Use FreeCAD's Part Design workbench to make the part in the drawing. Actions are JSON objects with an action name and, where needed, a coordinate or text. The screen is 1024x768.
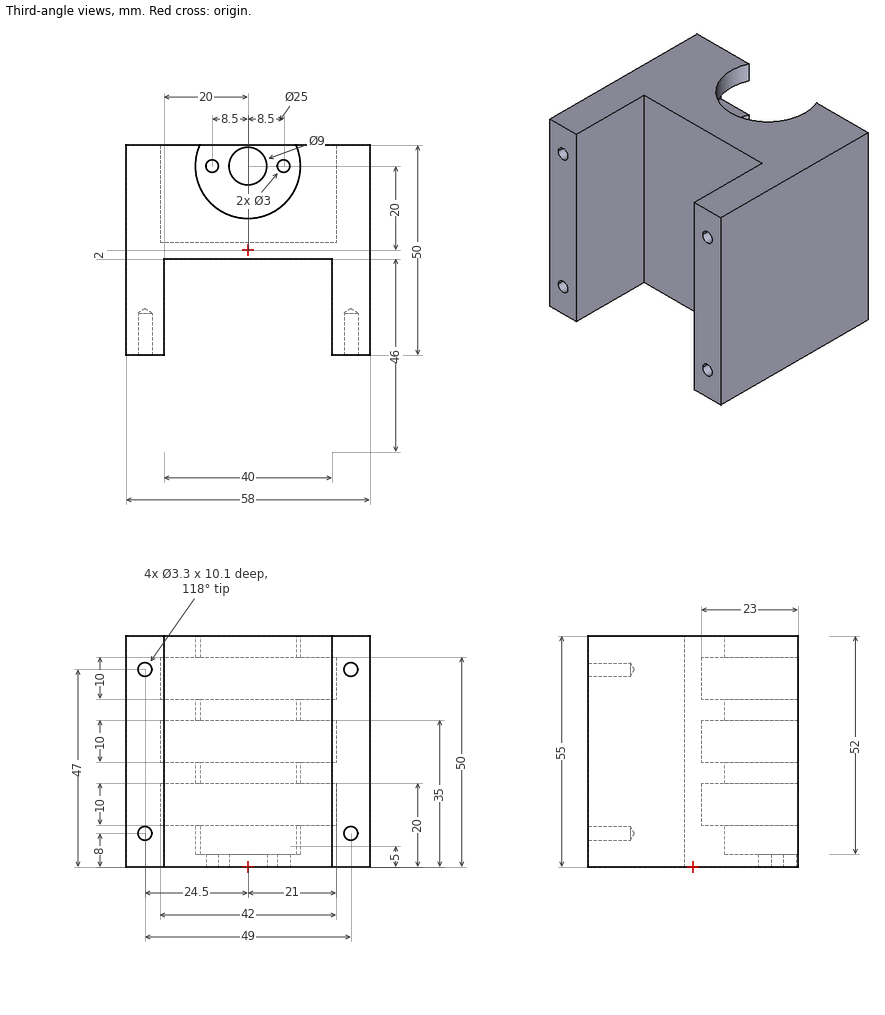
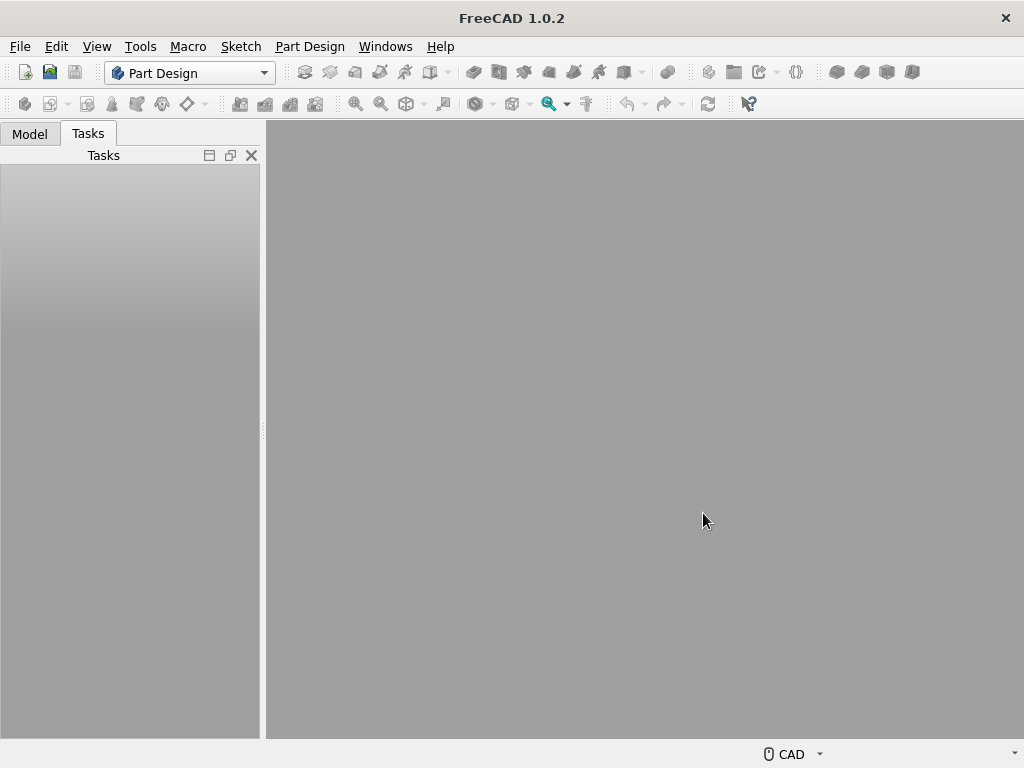
{"action": "left_click", "coordinate": [25, 72]}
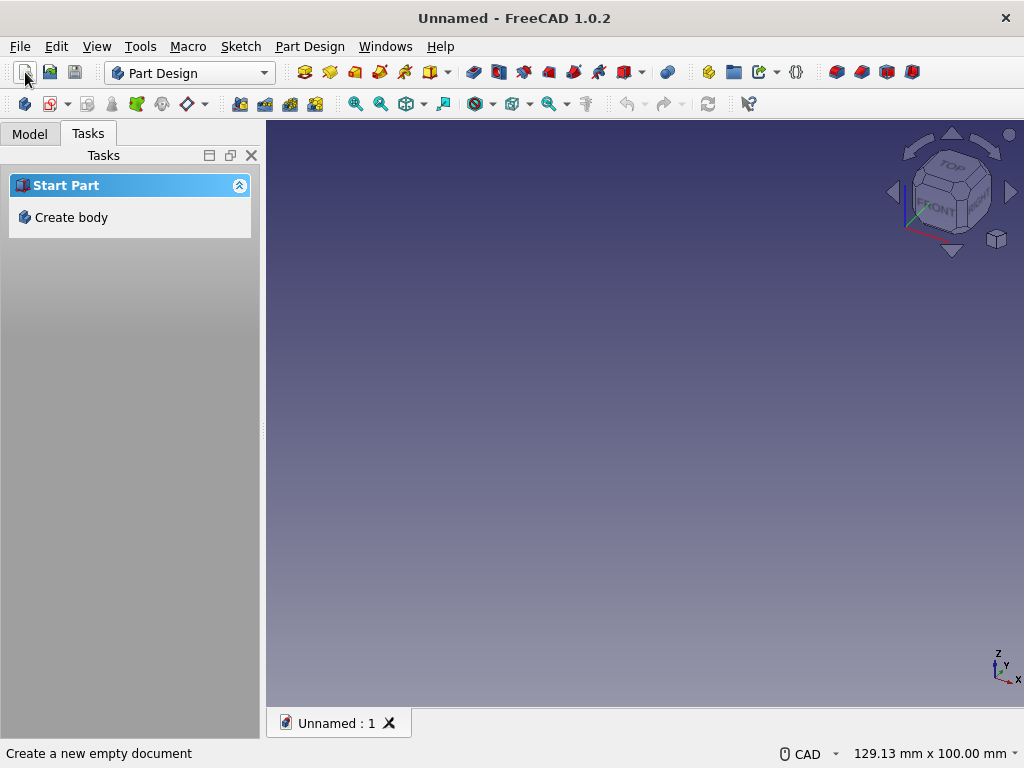
{"action": "left_click", "coordinate": [50, 104]}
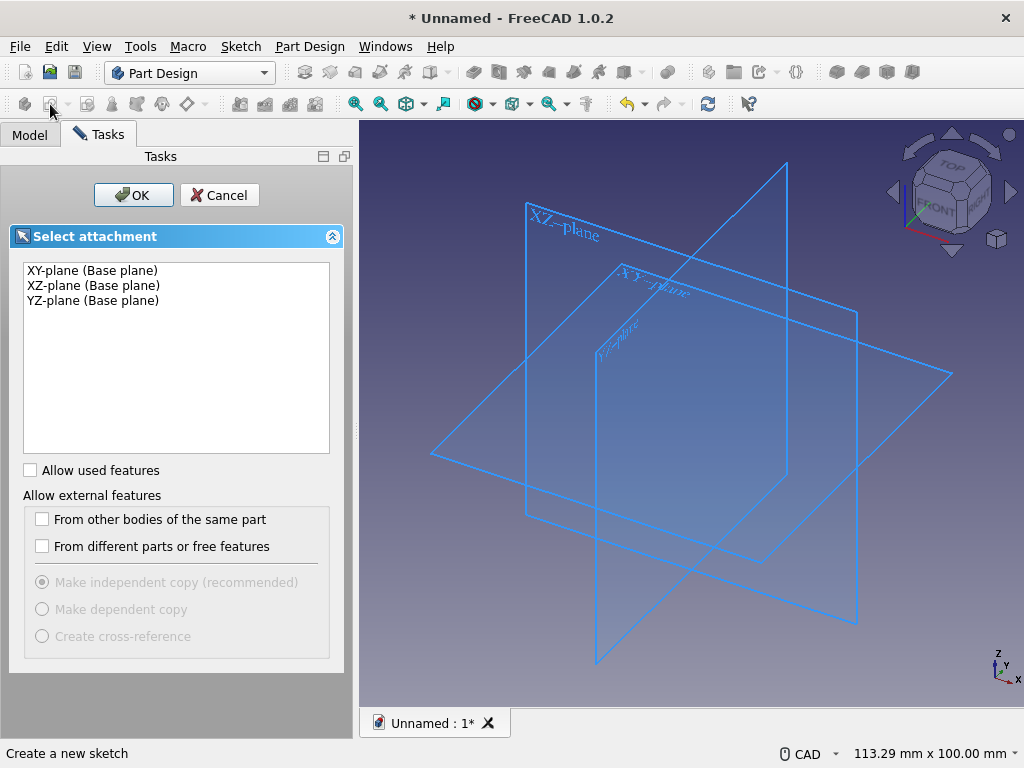
{"action": "left_click", "coordinate": [84, 270]}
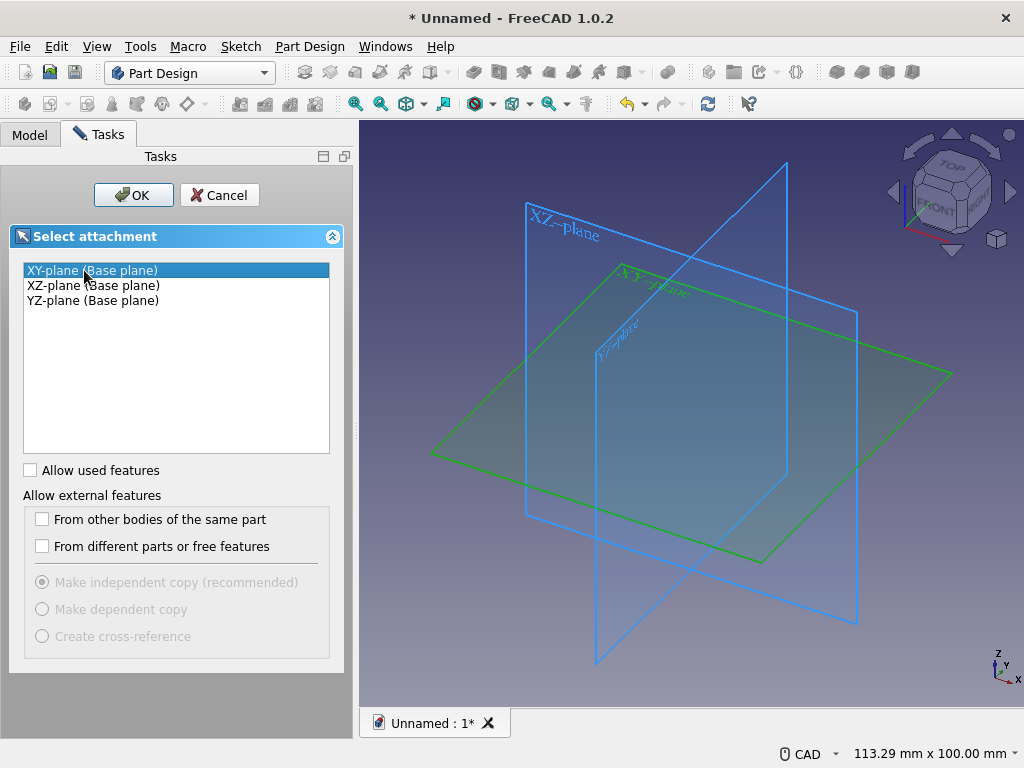
{"action": "left_click", "coordinate": [134, 195]}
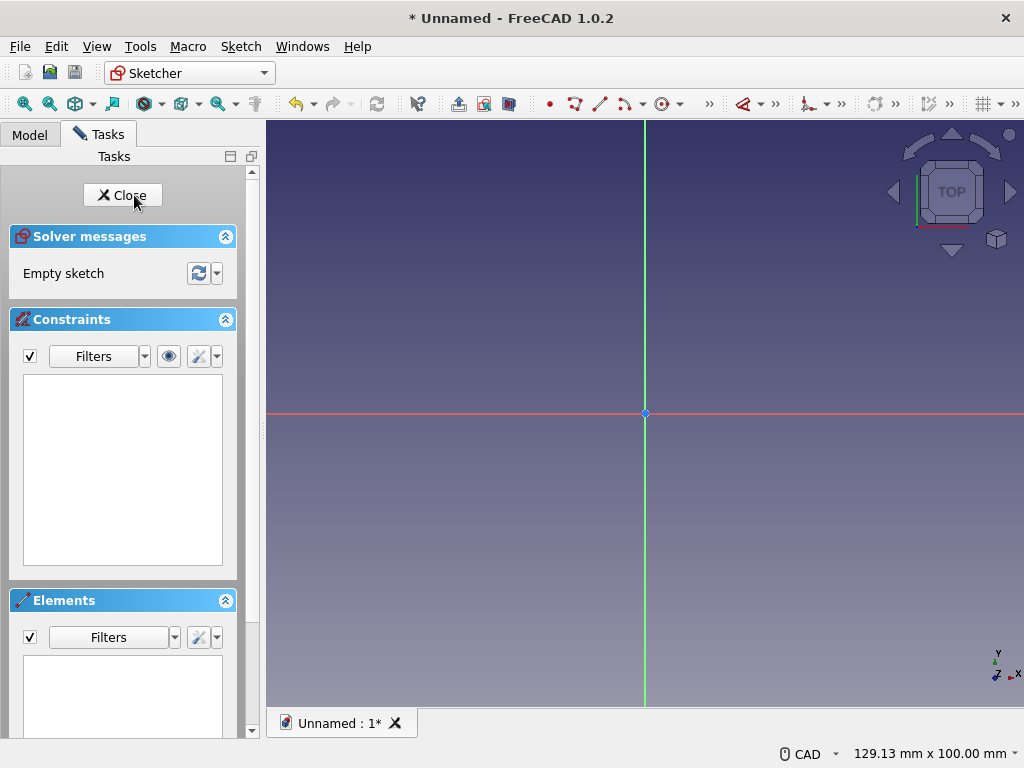
{"action": "key", "text": "g v"}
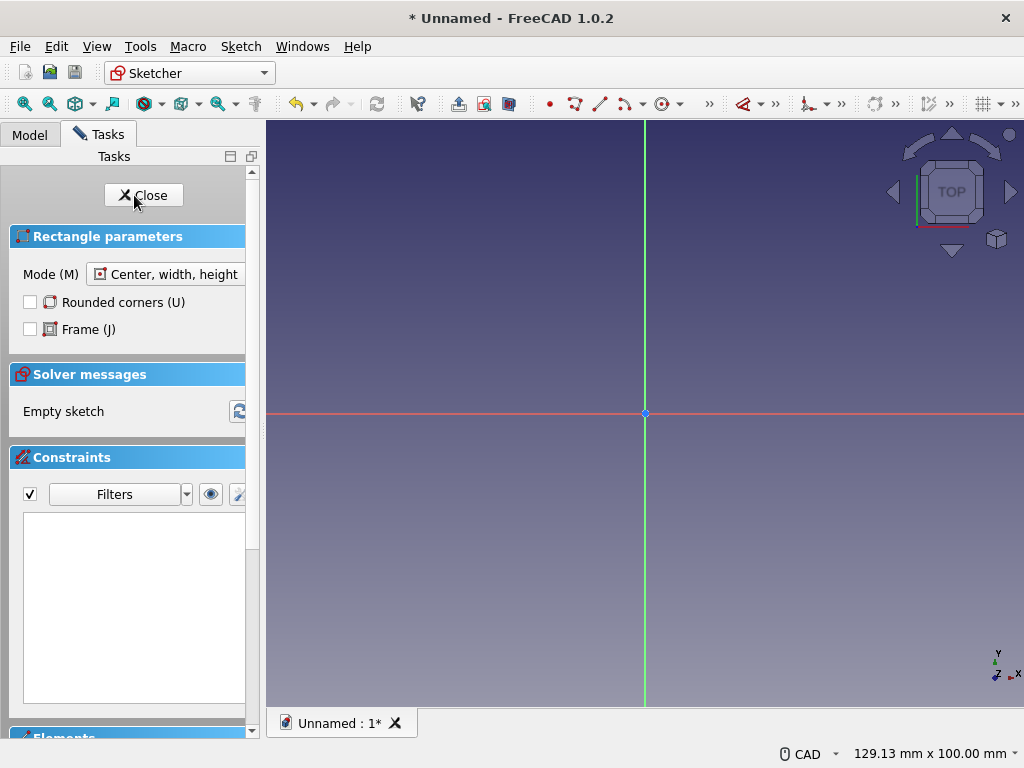
{"action": "left_click", "coordinate": [645, 414]}
{"action": "mouse_move", "coordinate": [815, 267]}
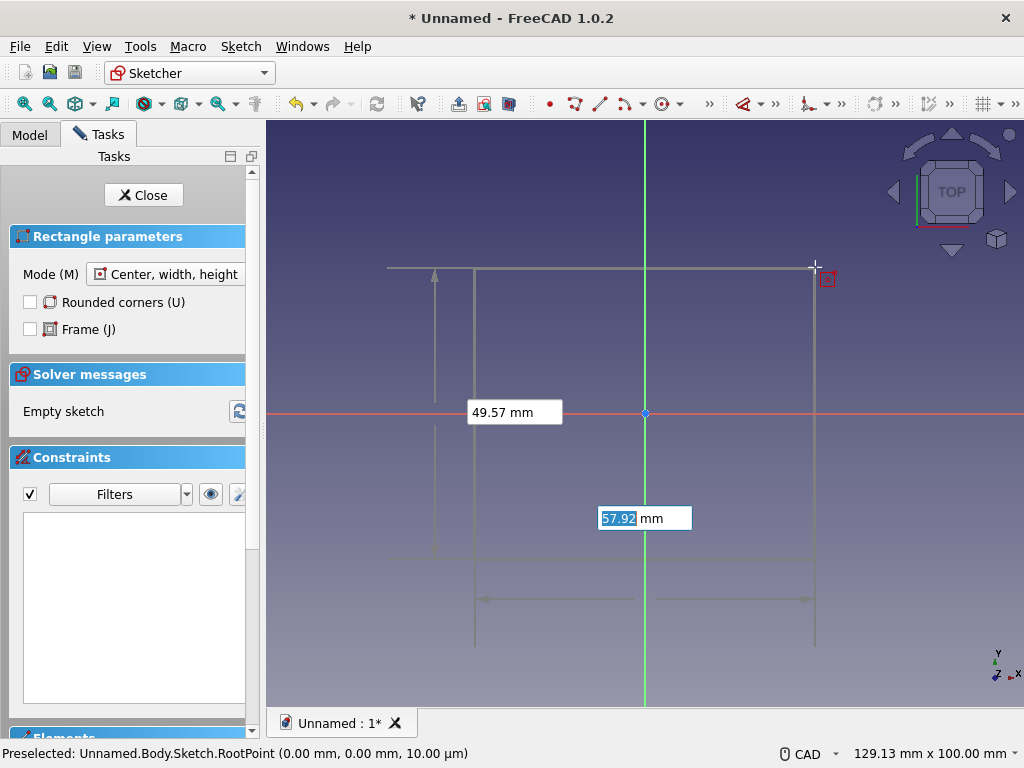
{"action": "type", "text": "58"}
{"action": "key", "text": "Tab"}
{"action": "type", "text": "50"}
{"action": "key", "text": "Return"}
{"action": "key", "text": "Escape"}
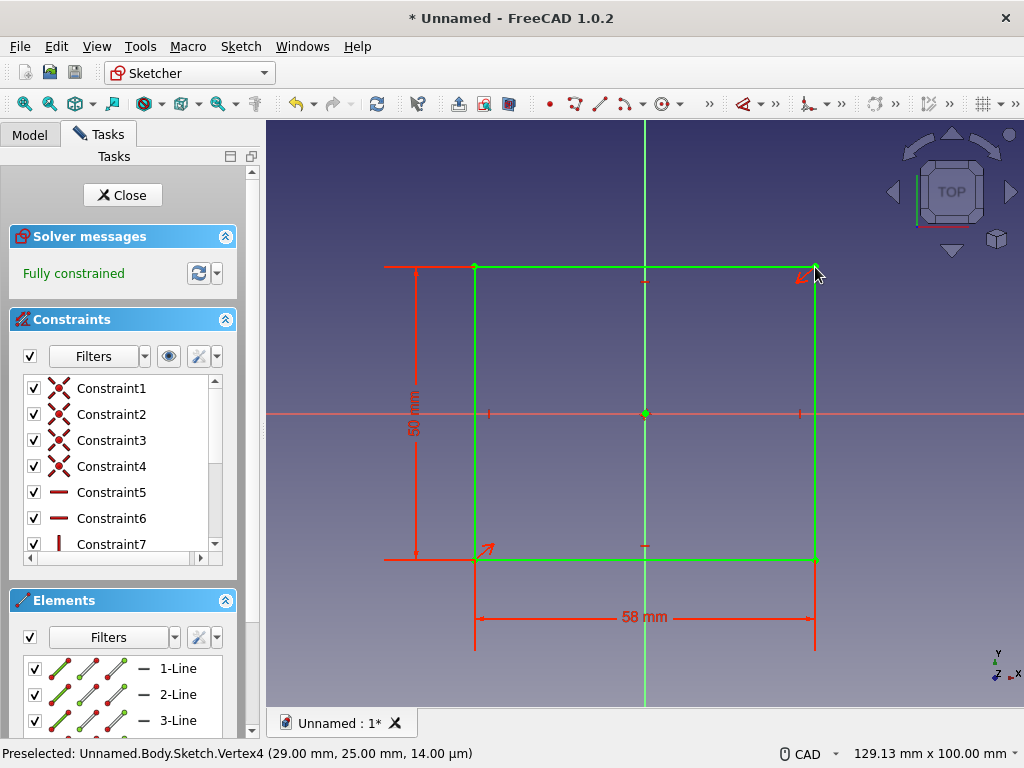
{"action": "left_click", "coordinate": [123, 195]}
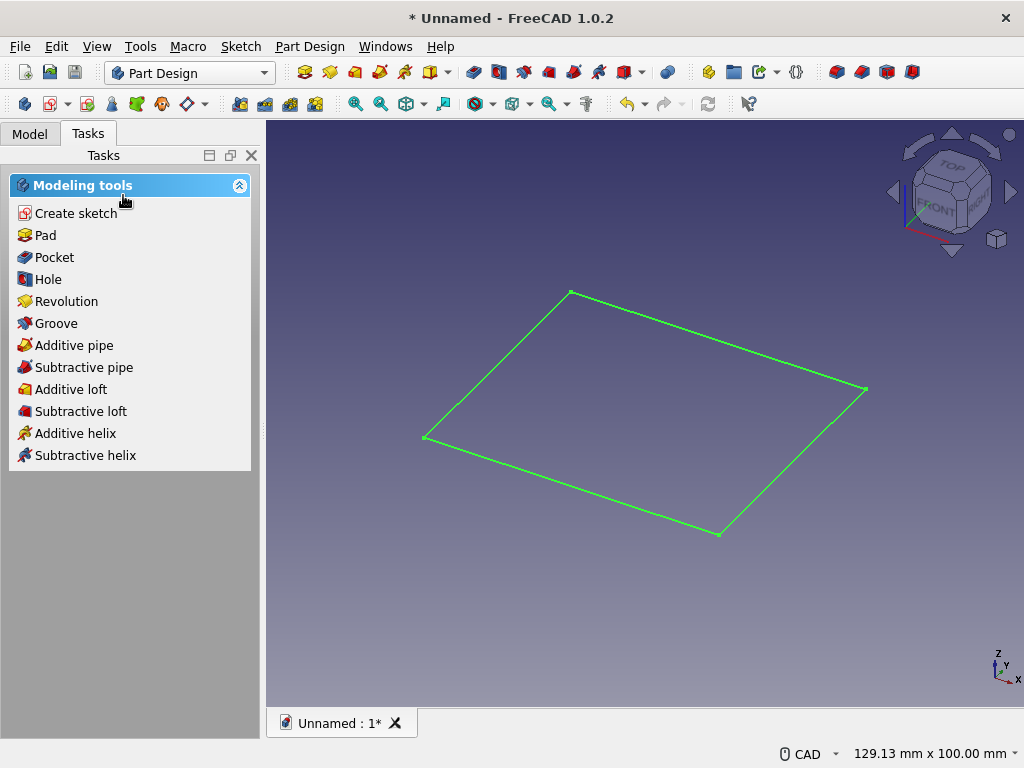
{"action": "left_click", "coordinate": [305, 72]}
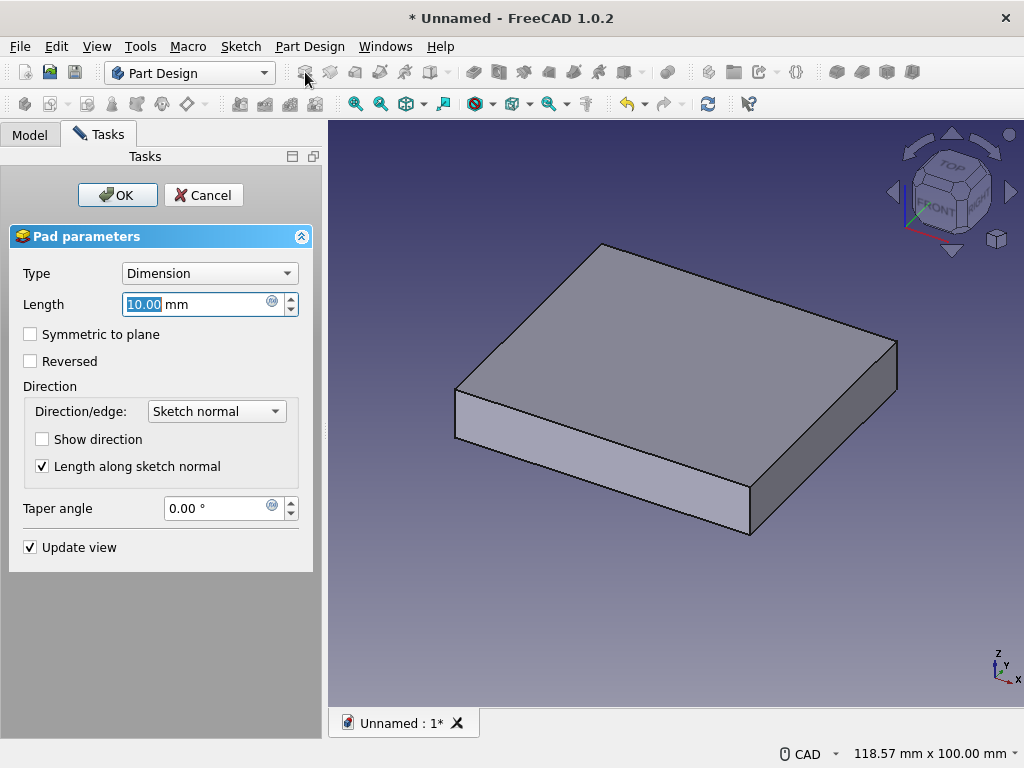
{"action": "type", "text": "55"}
{"action": "key", "text": "Tab"}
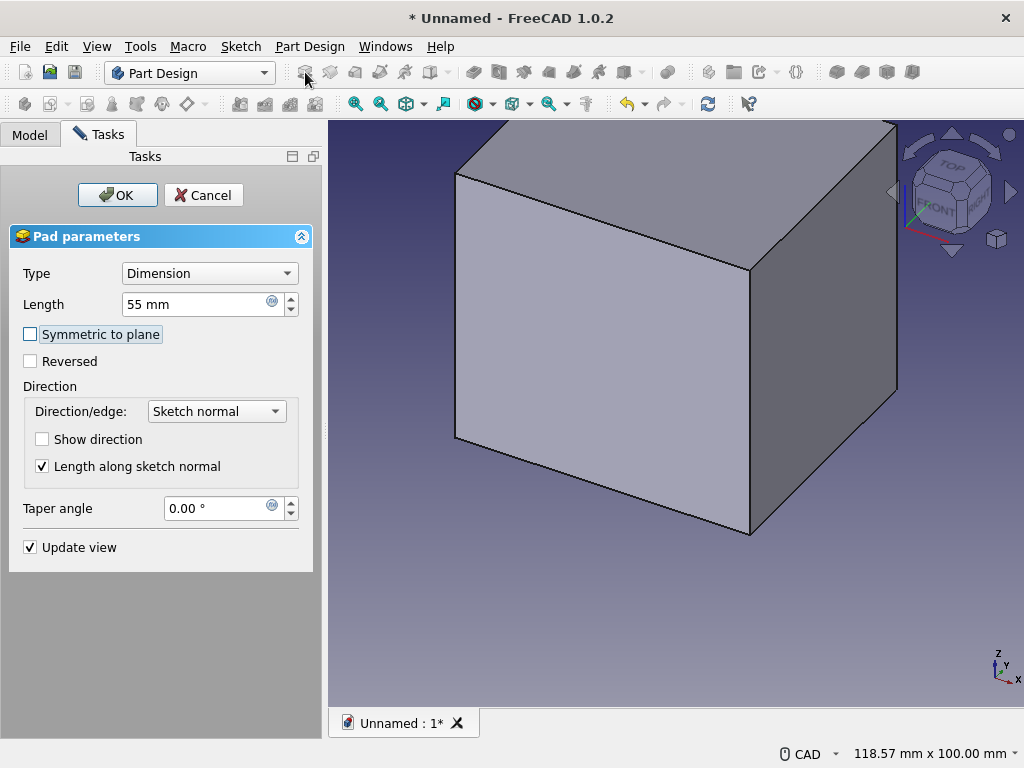
{"action": "left_click", "coordinate": [118, 195]}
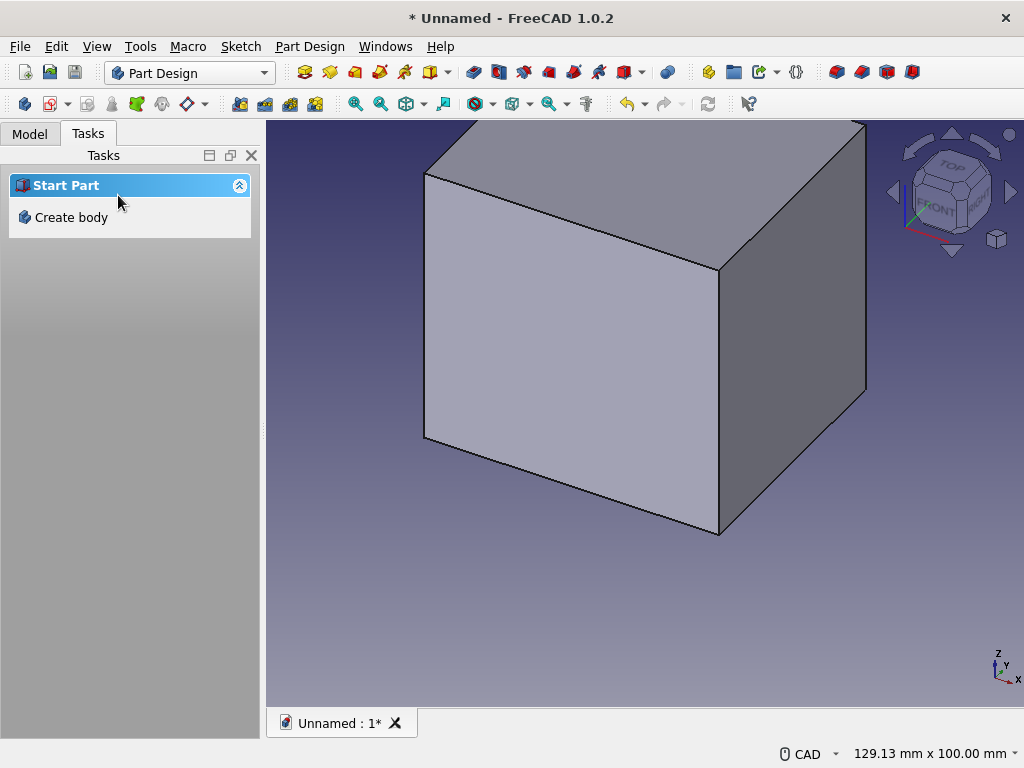
{"action": "left_click", "coordinate": [356, 104]}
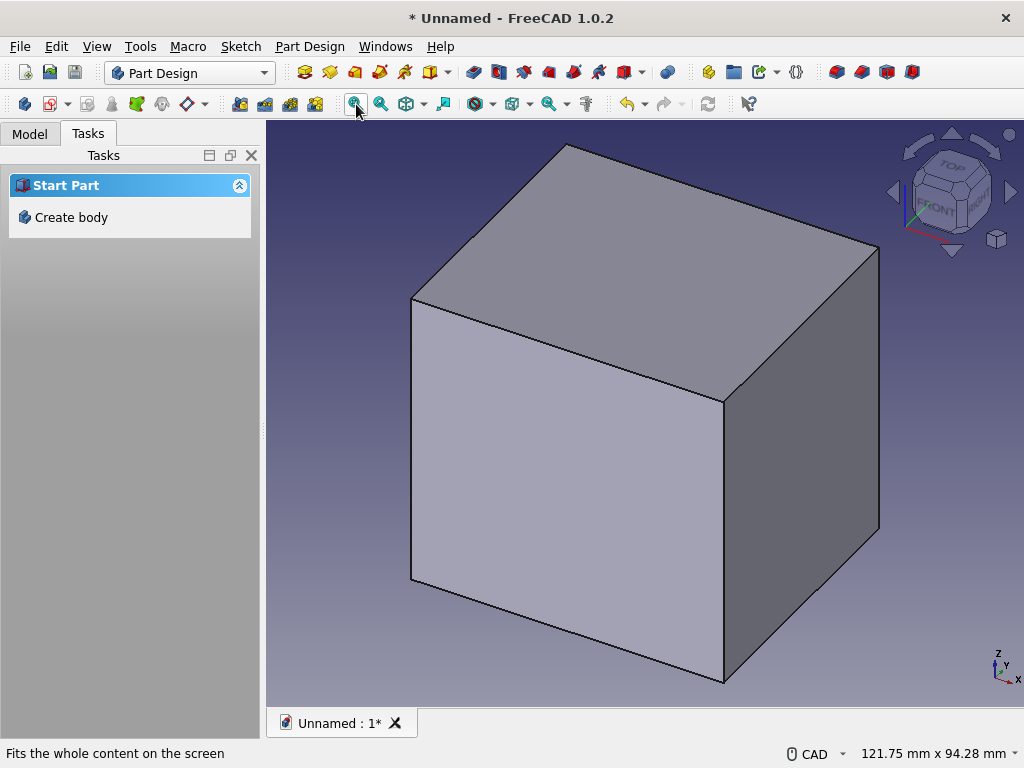
{"action": "key", "text": "5"}